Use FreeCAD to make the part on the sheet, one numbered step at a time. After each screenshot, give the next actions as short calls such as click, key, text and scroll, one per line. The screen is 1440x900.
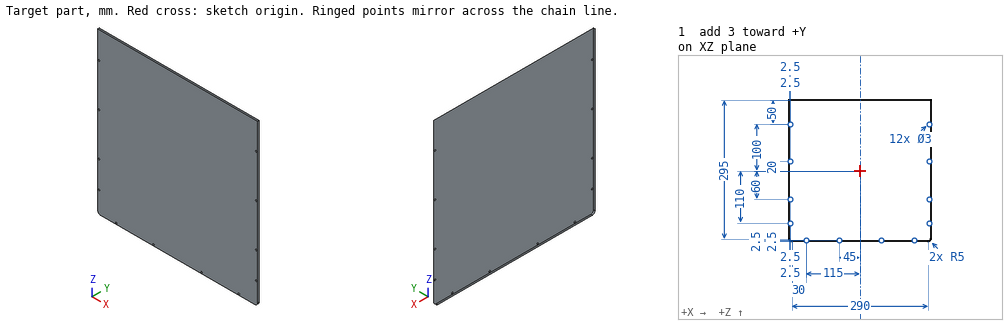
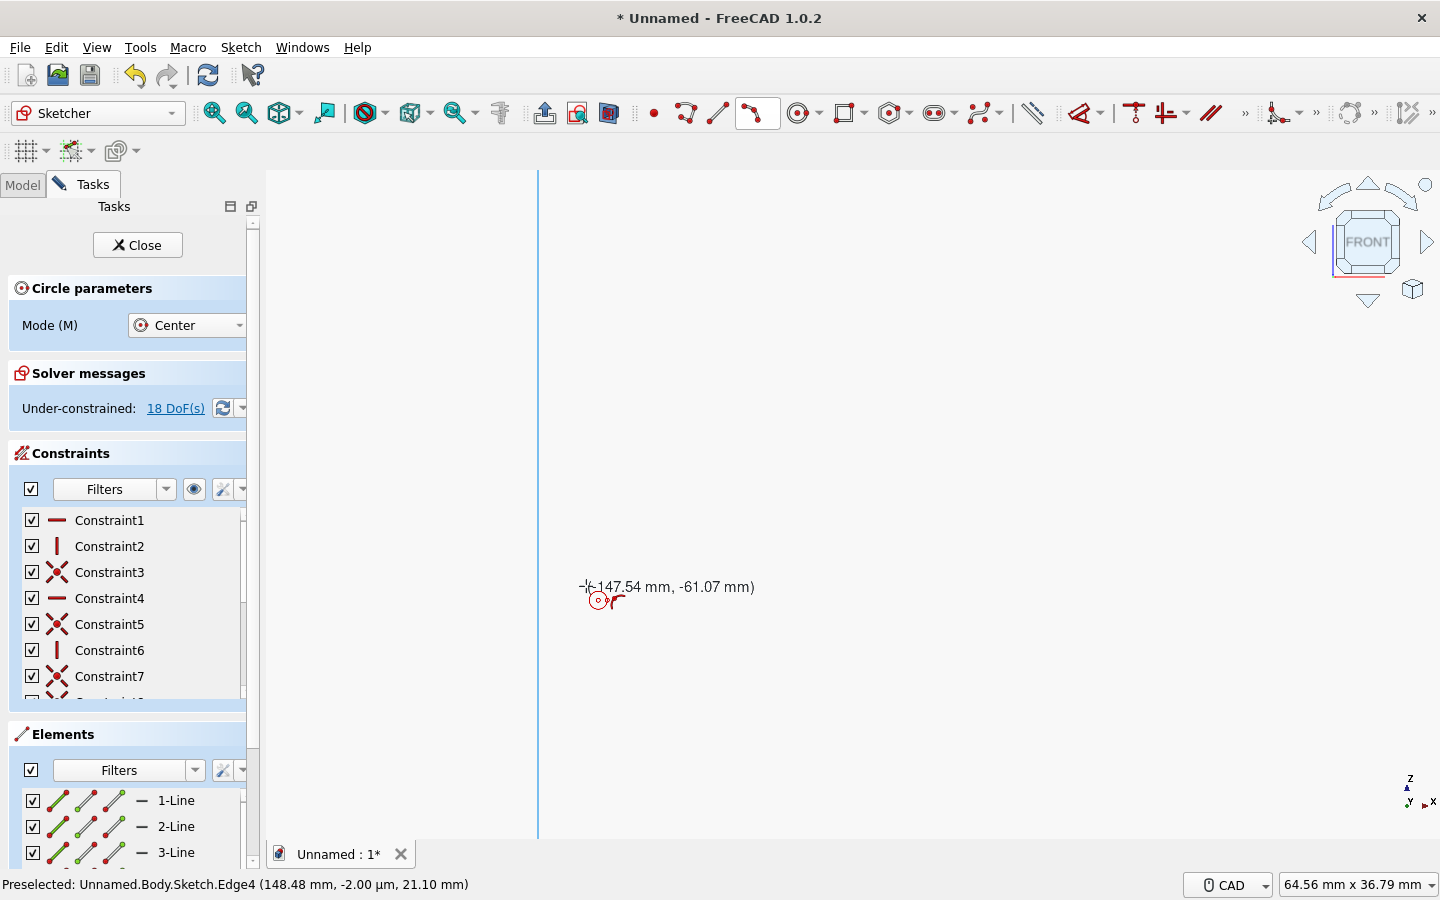
click(583, 572)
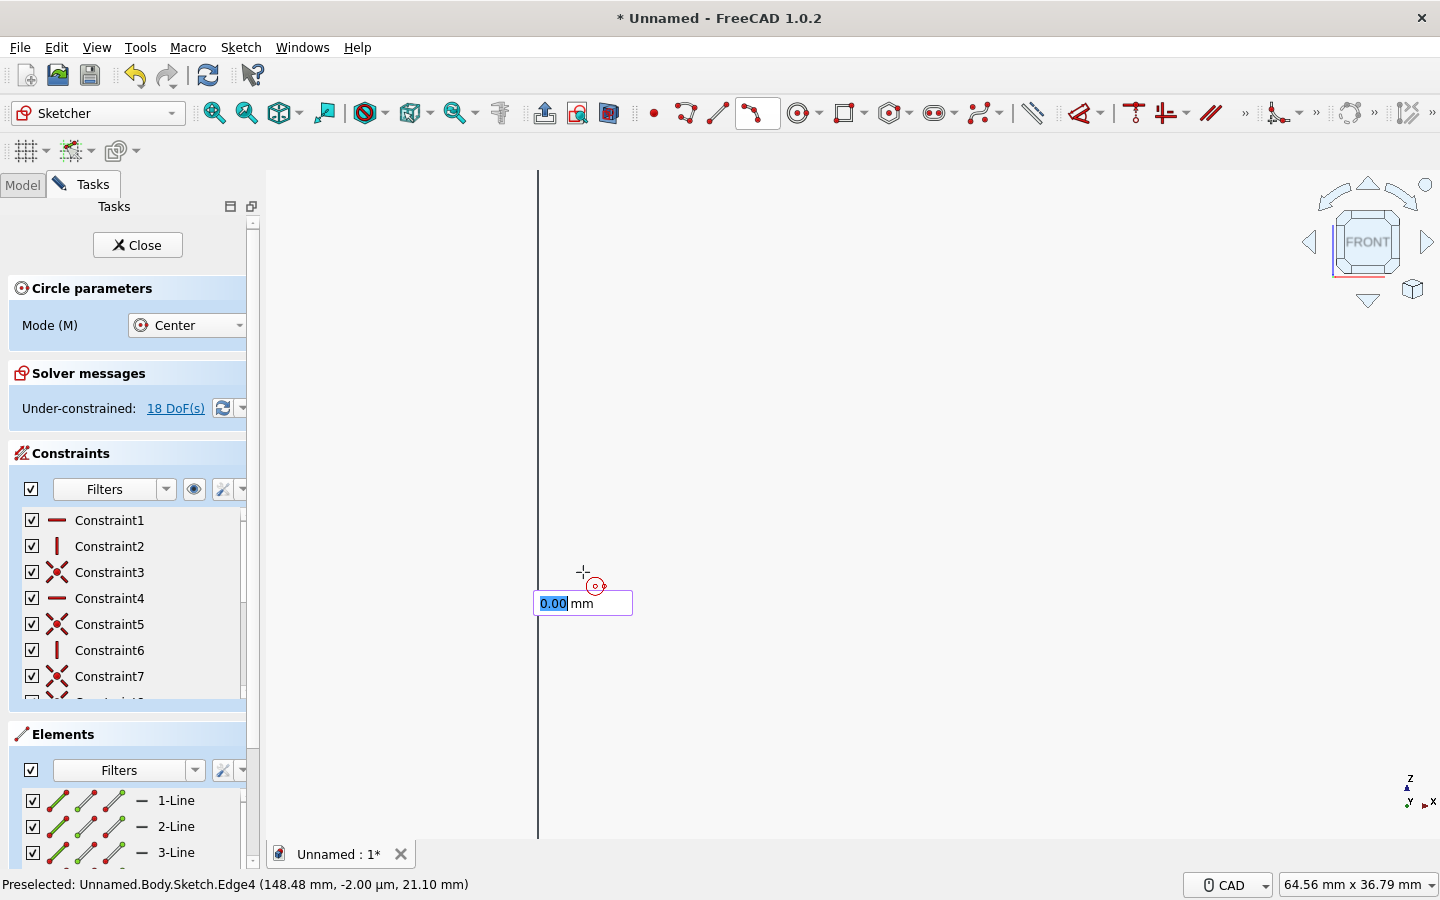
scroll(585, 587, down, 13)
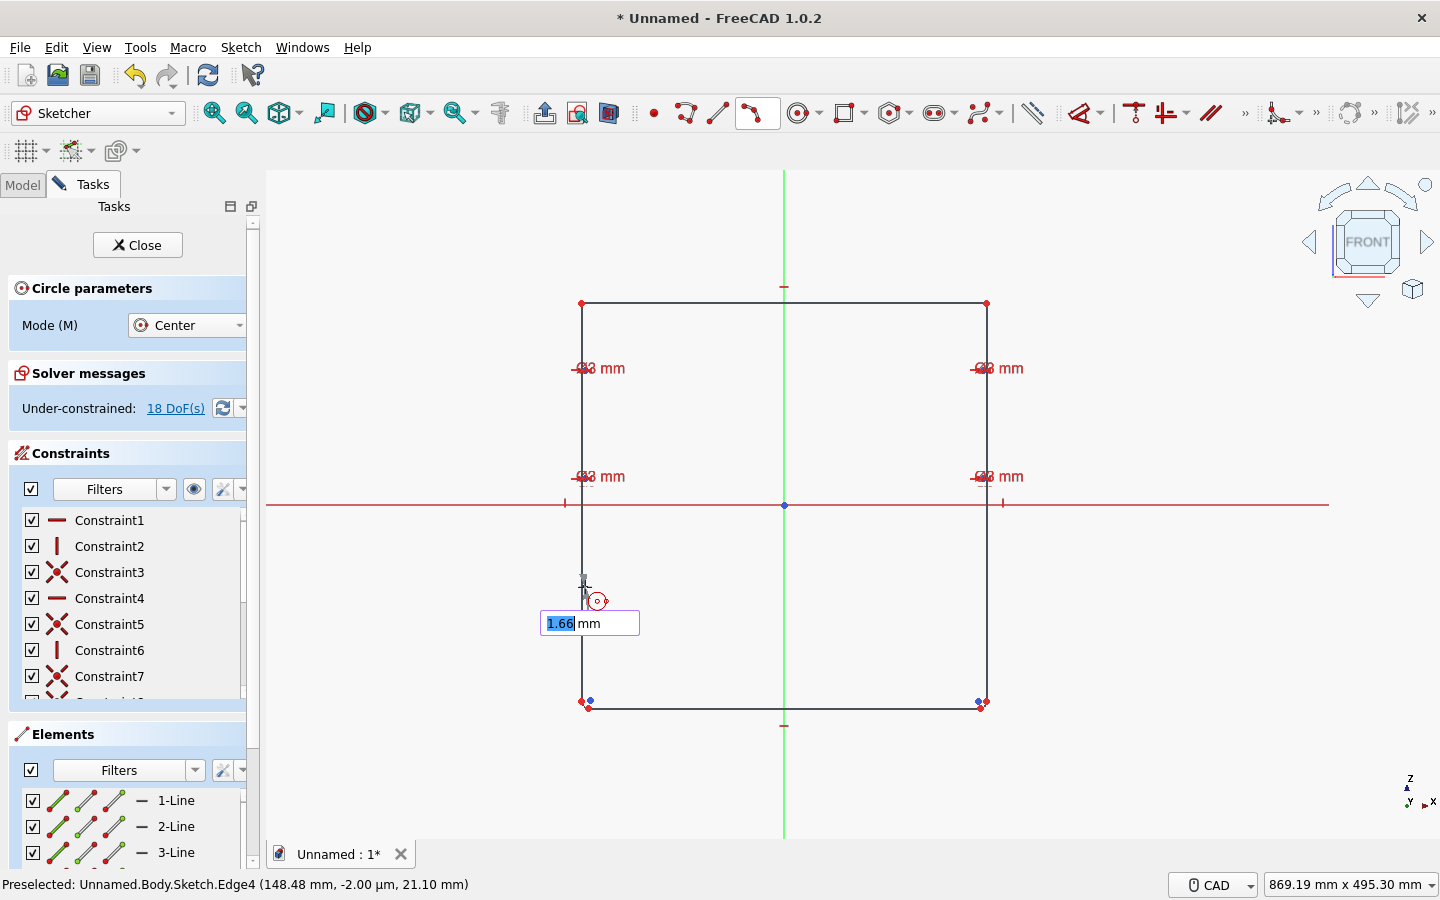
scroll(587, 585, up, 6)
move(585, 584)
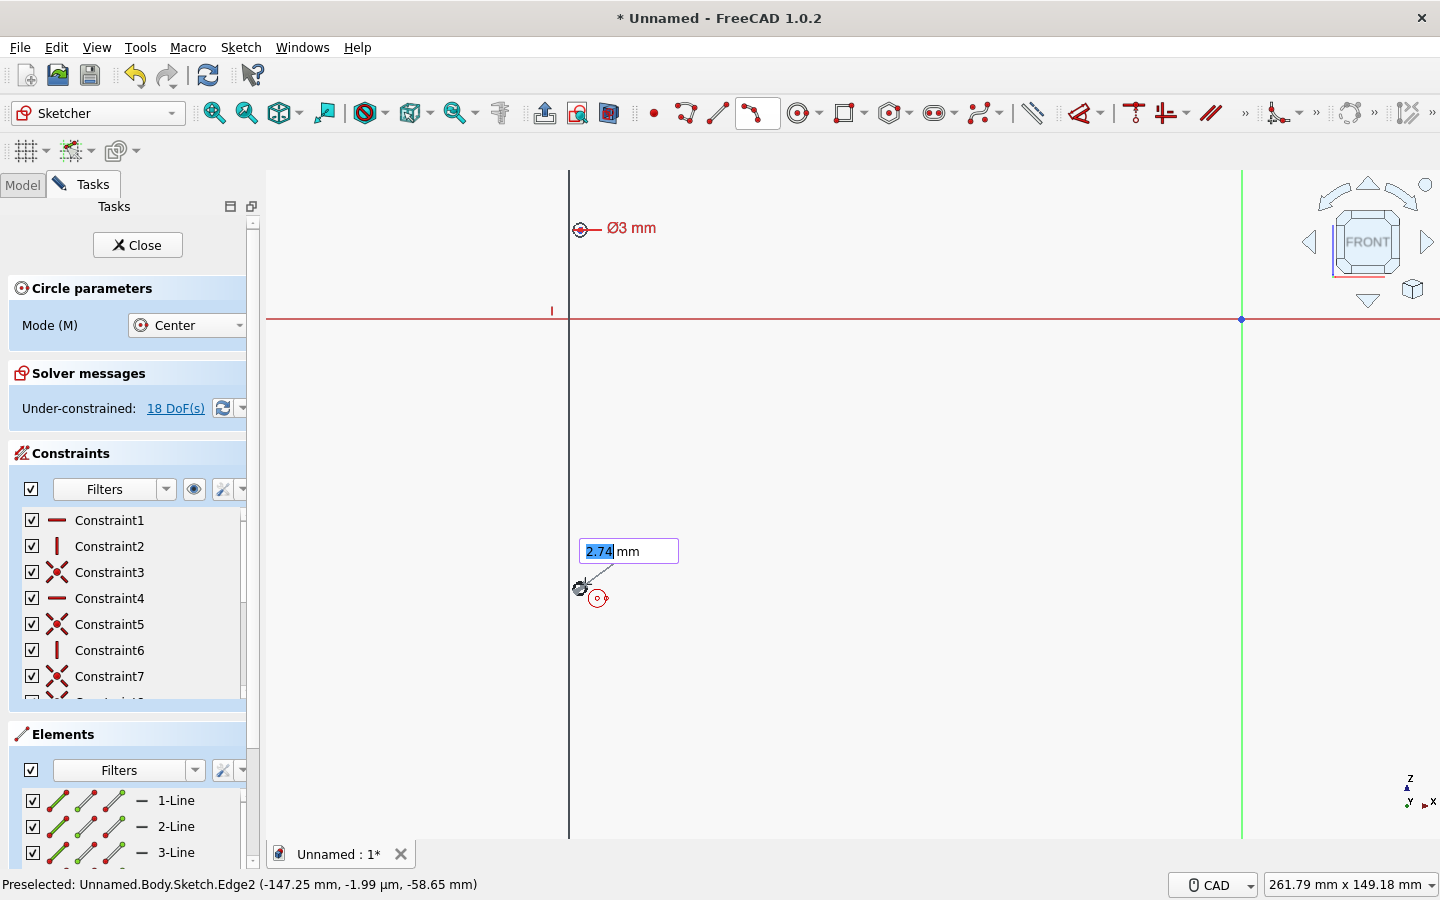
text(3)
key(Return)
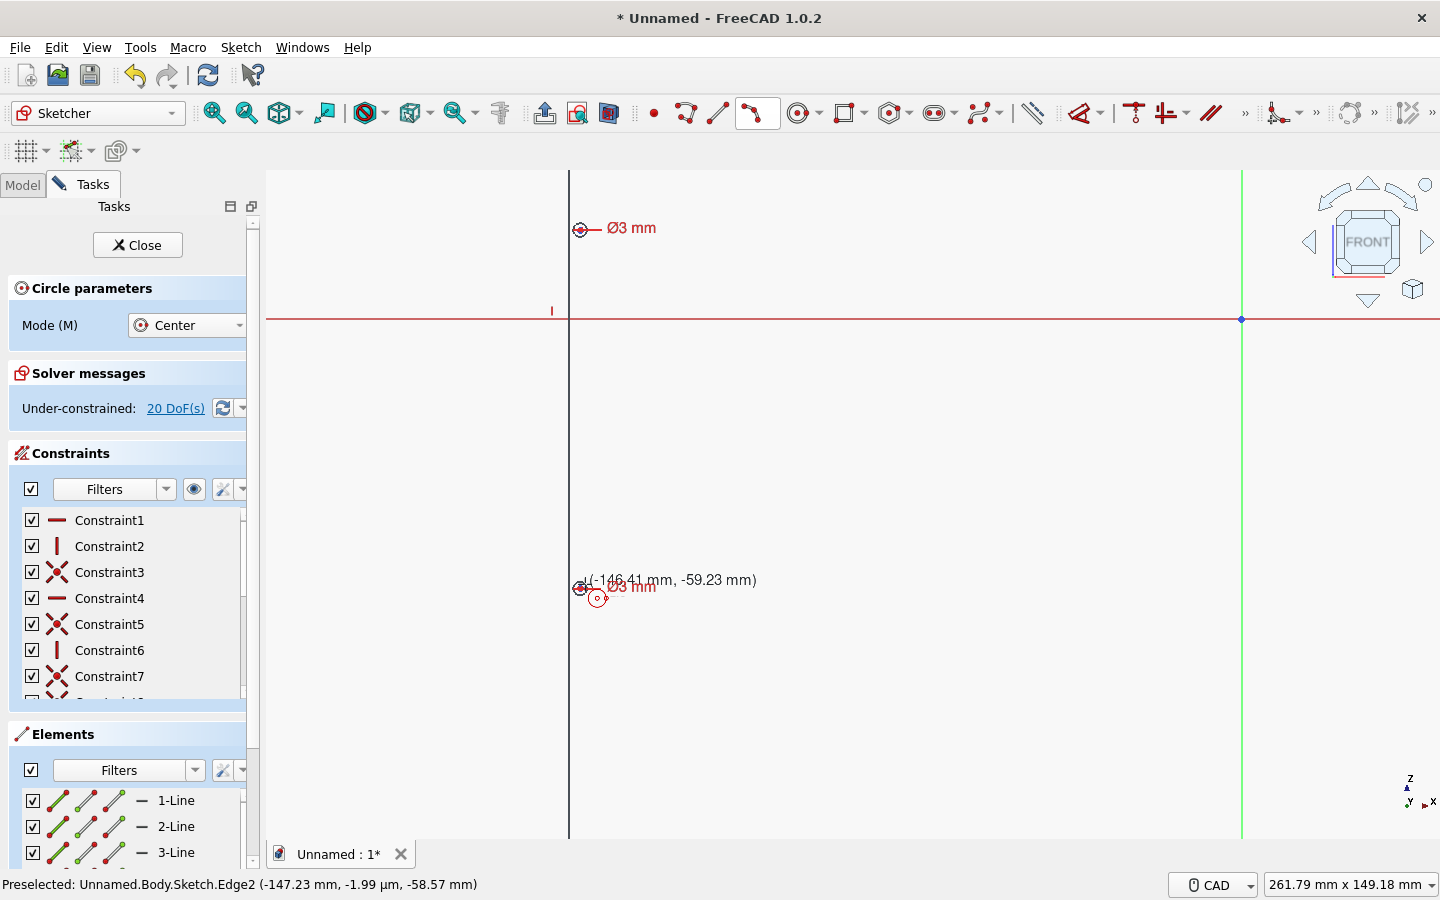
scroll(587, 584, down, 6)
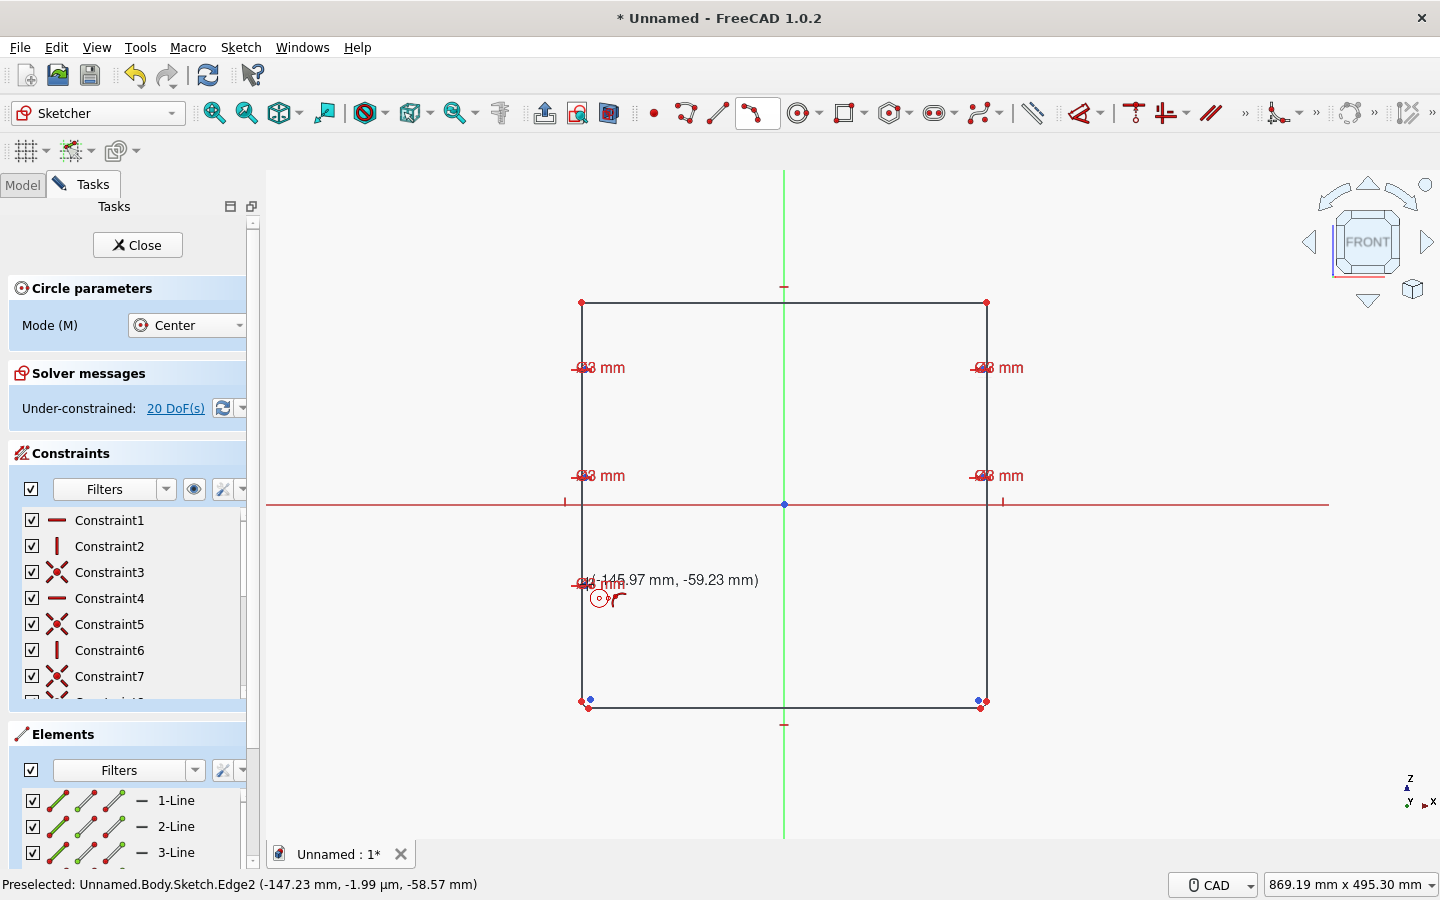
scroll(585, 653, up, 13)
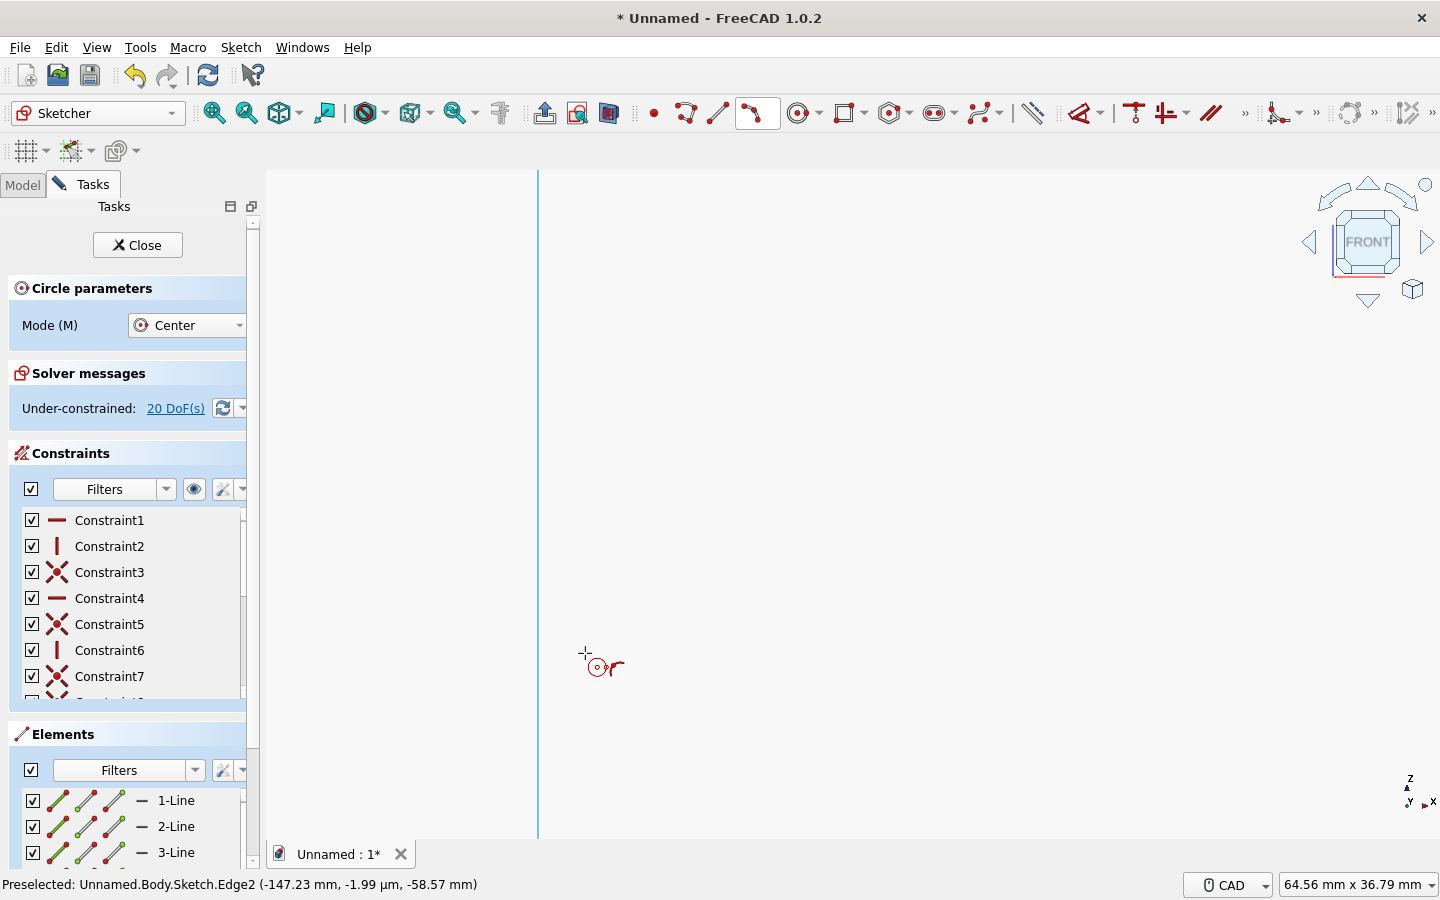
click(583, 648)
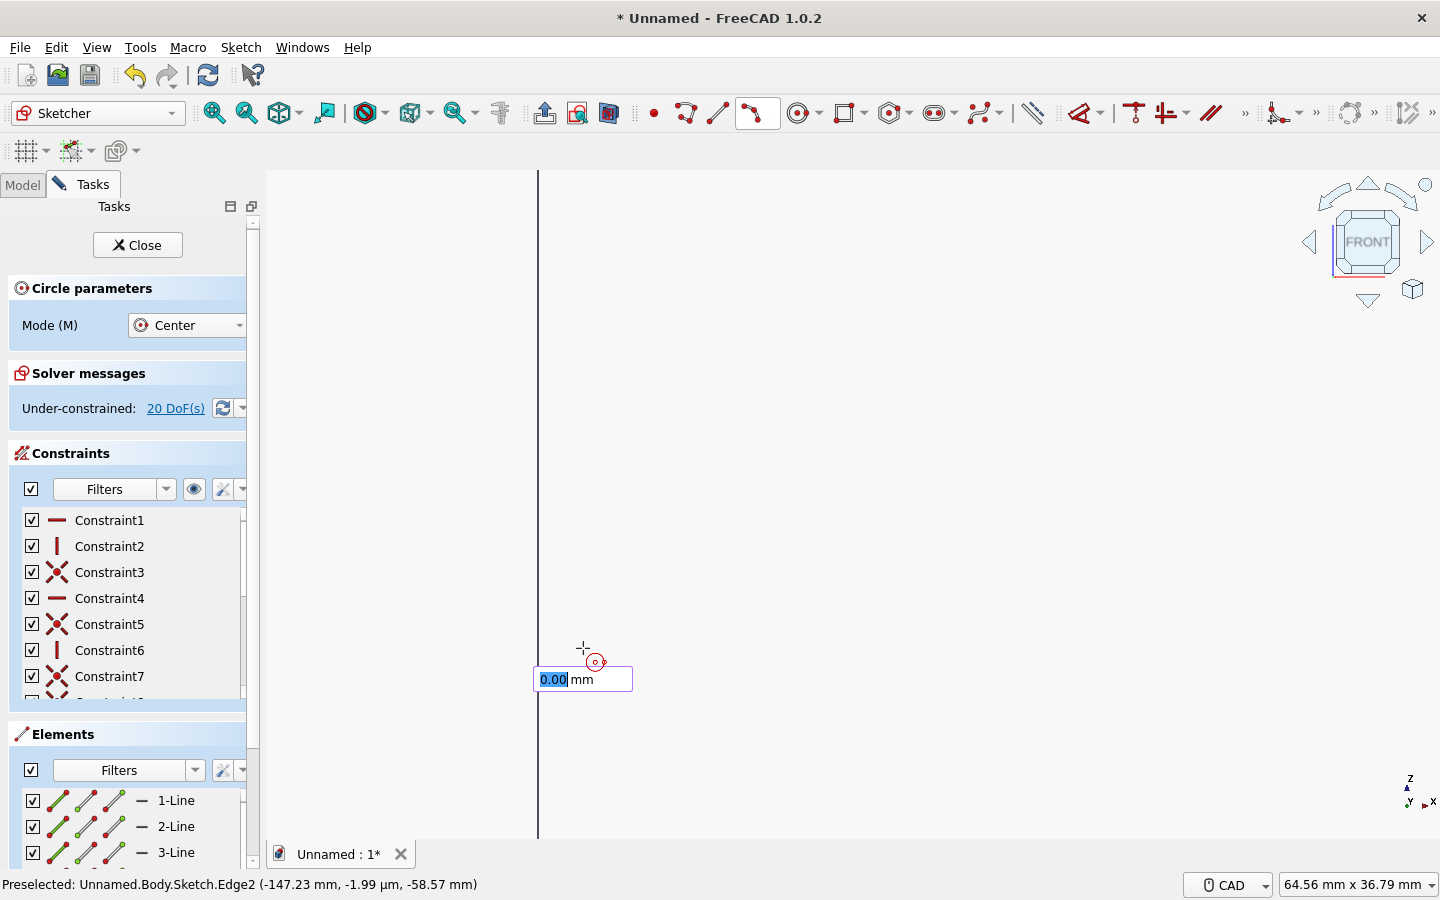
scroll(585, 653, down, 13)